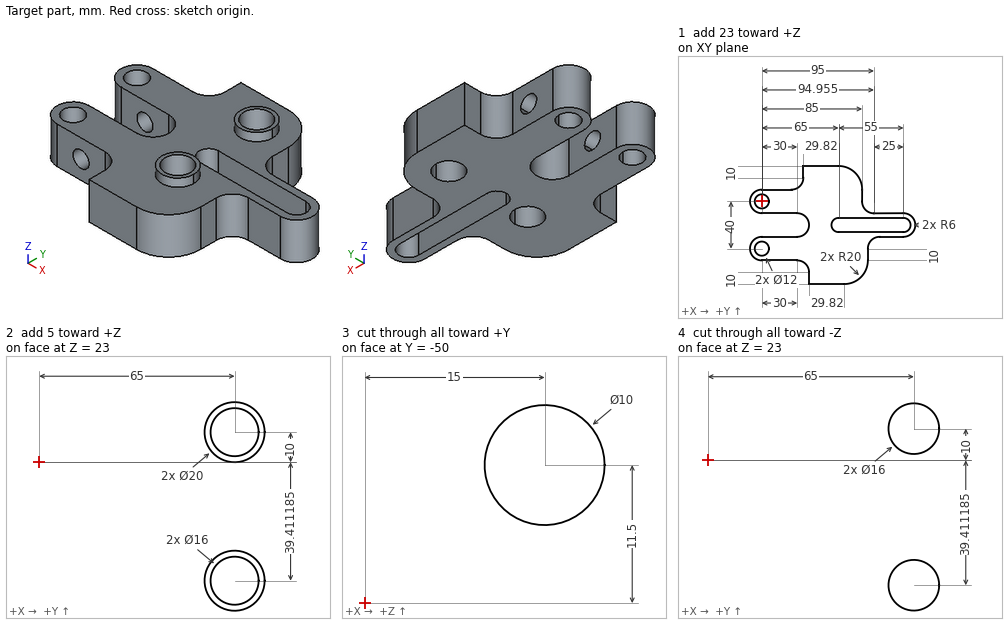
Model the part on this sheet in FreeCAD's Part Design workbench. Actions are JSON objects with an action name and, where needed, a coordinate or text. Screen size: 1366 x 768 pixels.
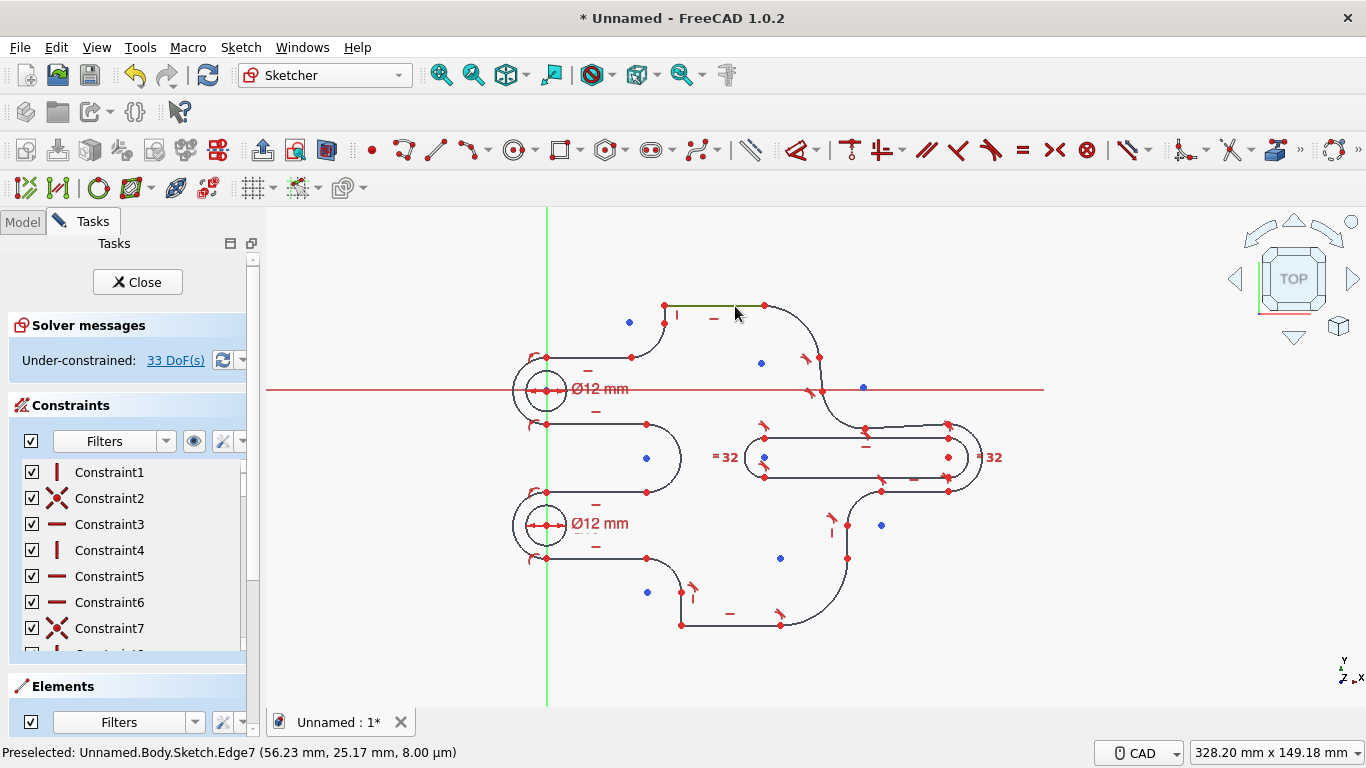
{"action": "left_click", "coordinate": [812, 334]}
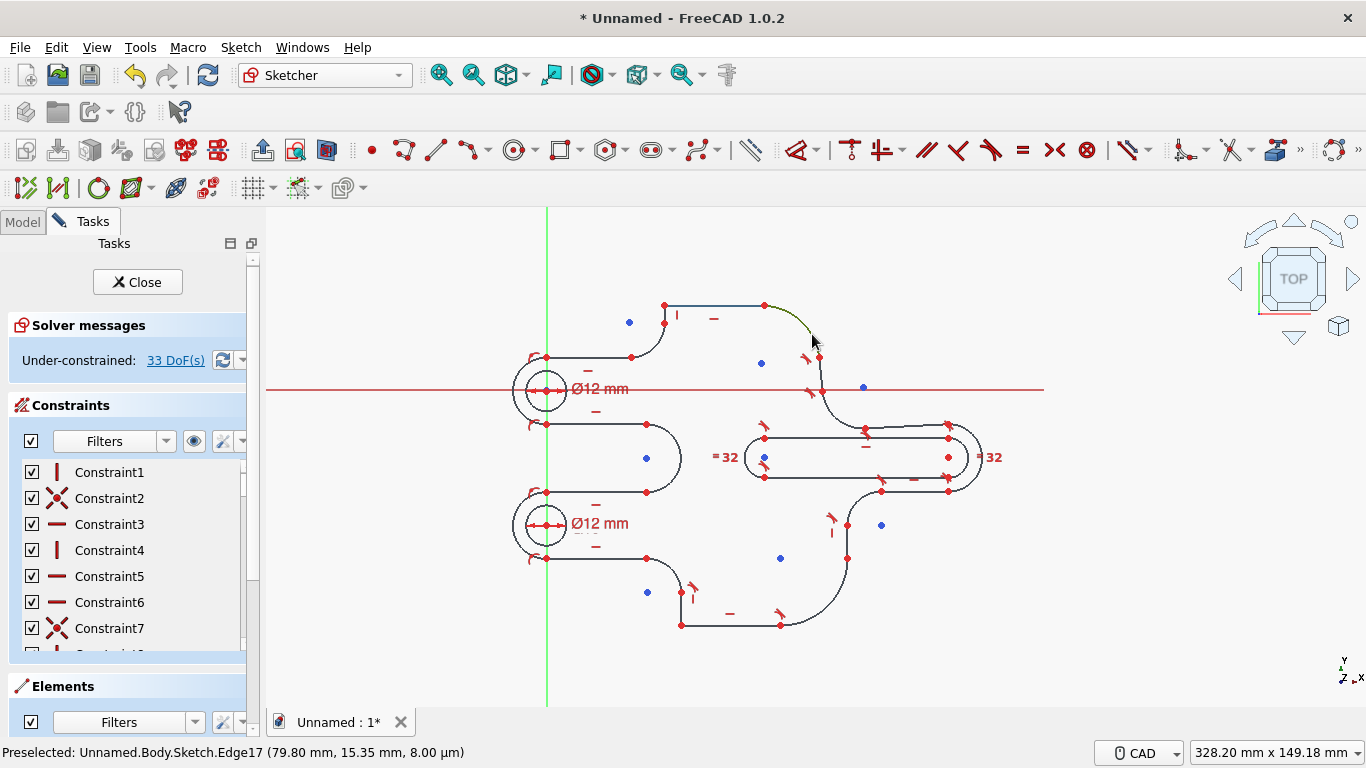
{"action": "left_click", "coordinate": [992, 150]}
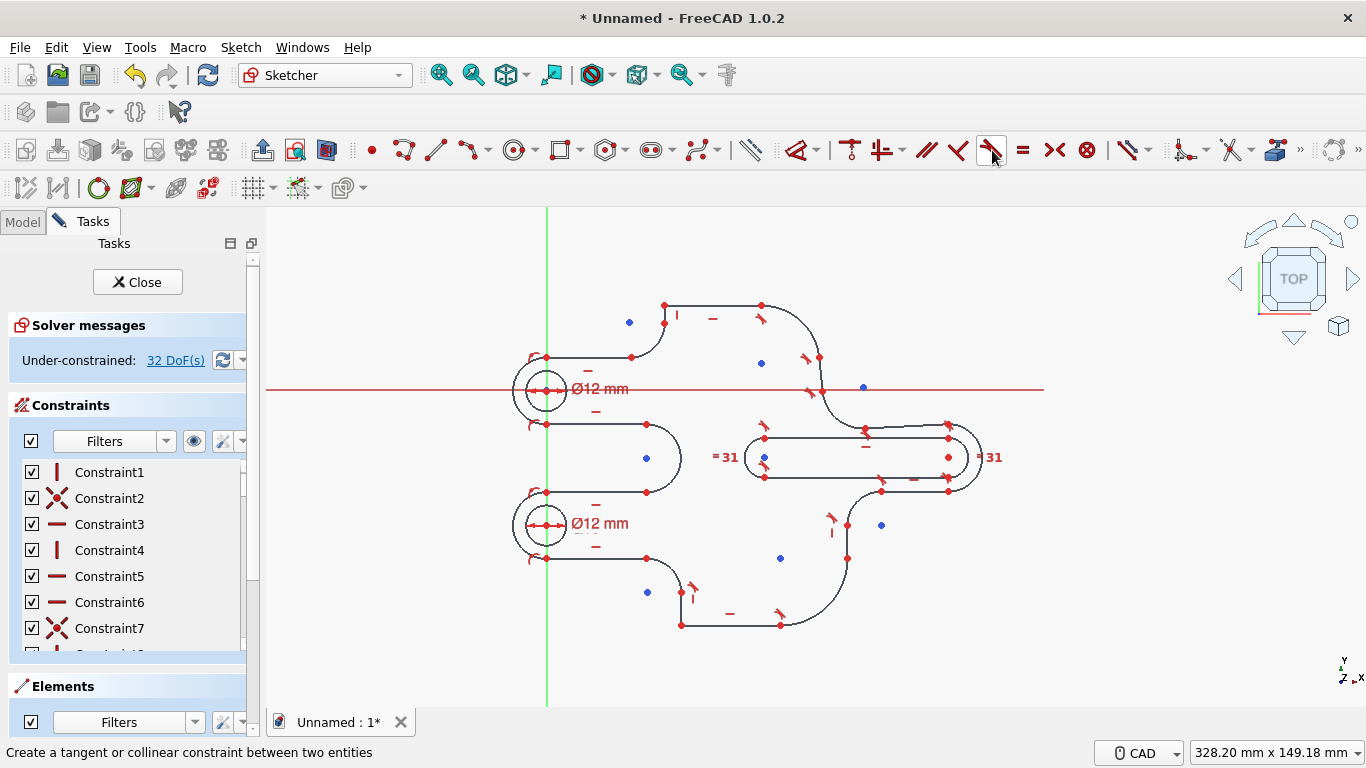
{"action": "scroll", "coordinate": [665, 315], "scroll_direction": "up", "scroll_amount": 3}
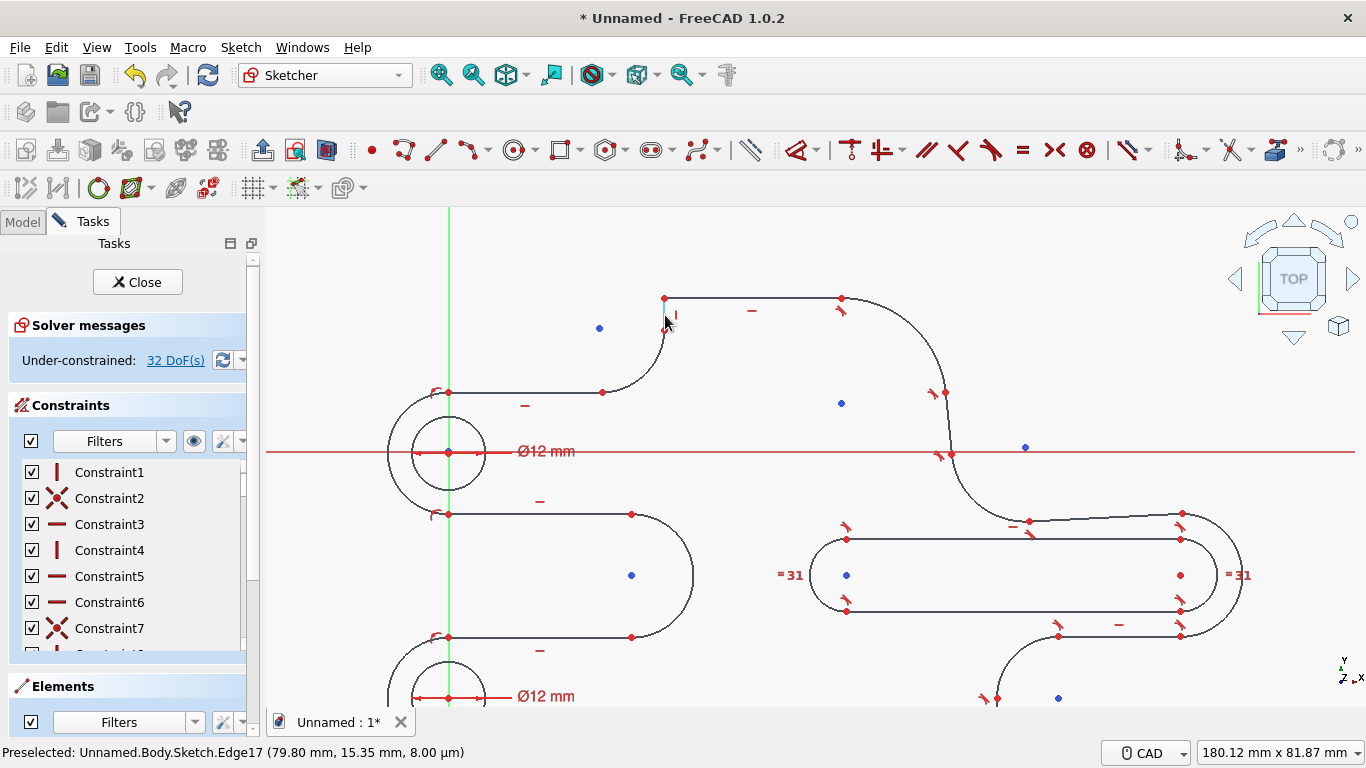
{"action": "left_click", "coordinate": [664, 315]}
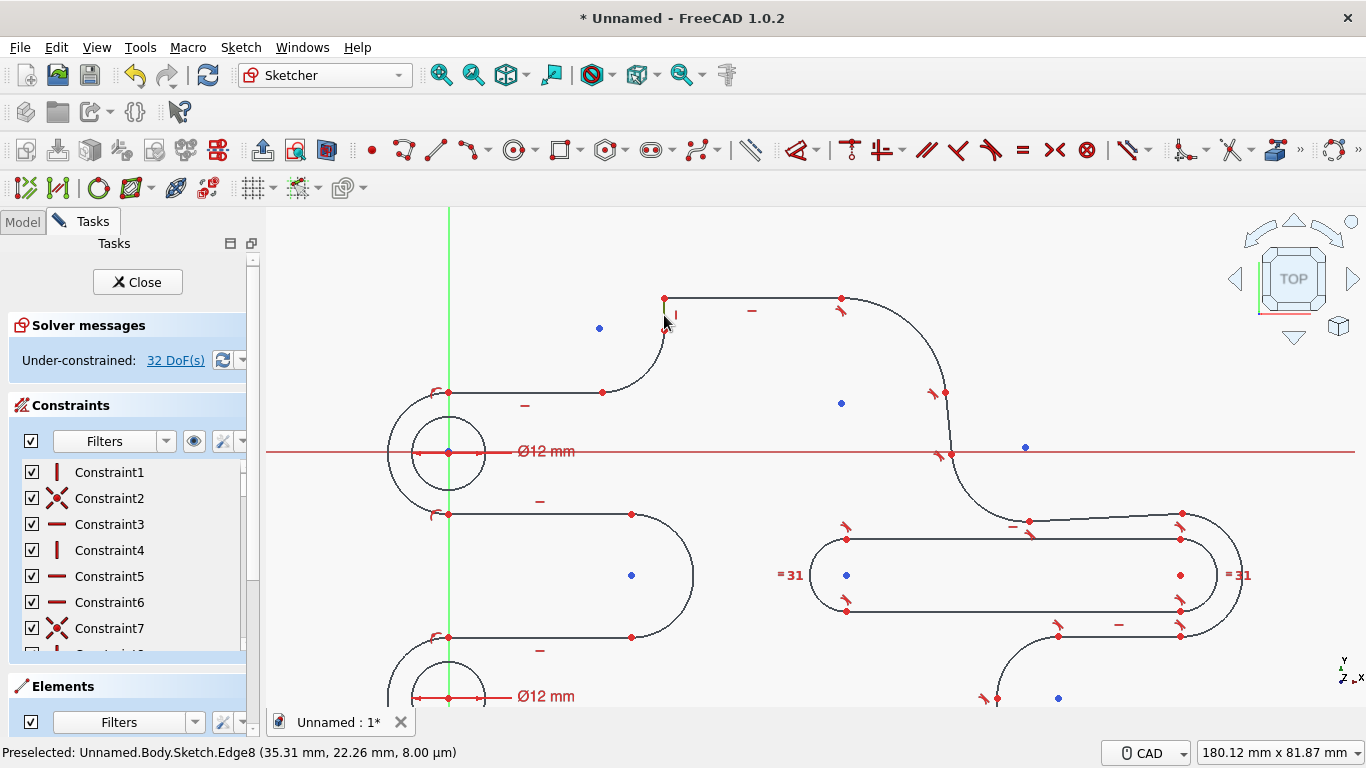
{"action": "left_click", "coordinate": [630, 385]}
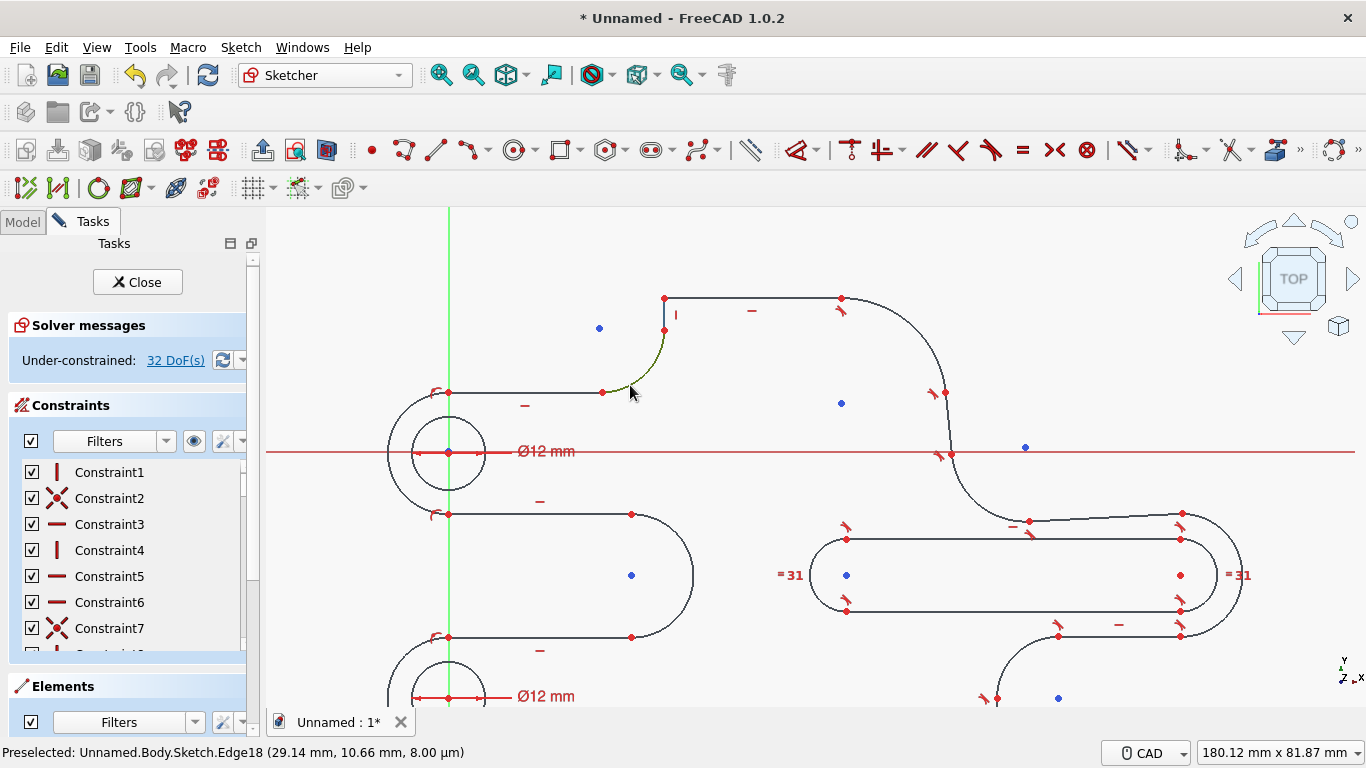
{"action": "left_click", "coordinate": [992, 150]}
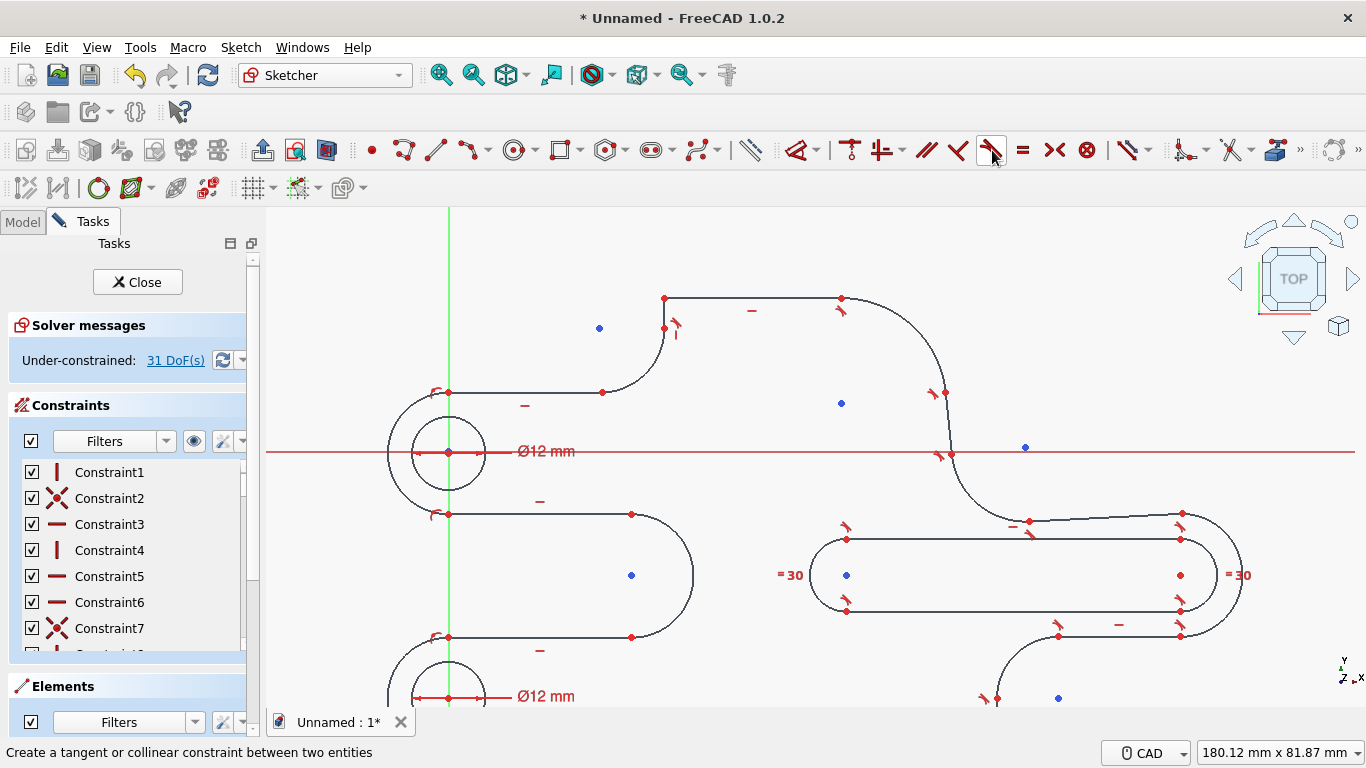
{"action": "left_click", "coordinate": [557, 393]}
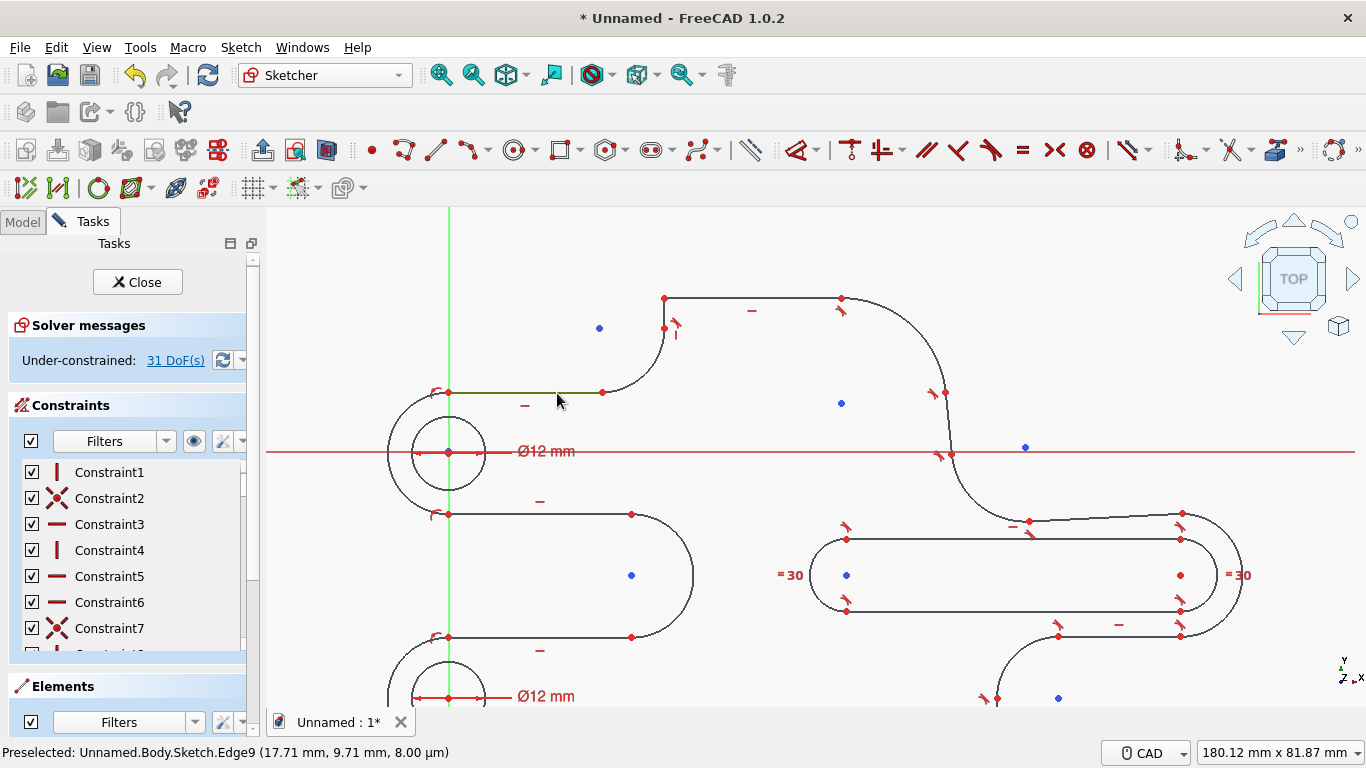
{"action": "left_click", "coordinate": [631, 385]}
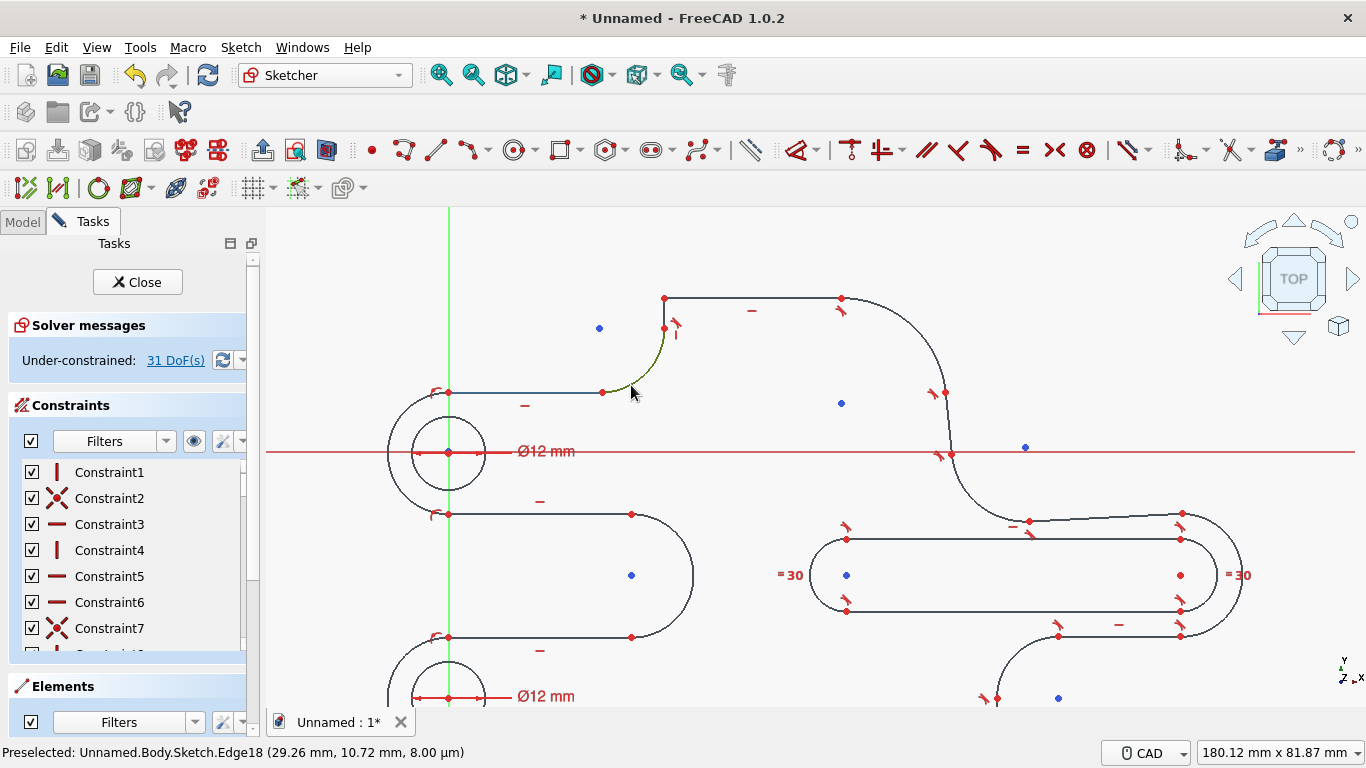
{"action": "key", "text": "t"}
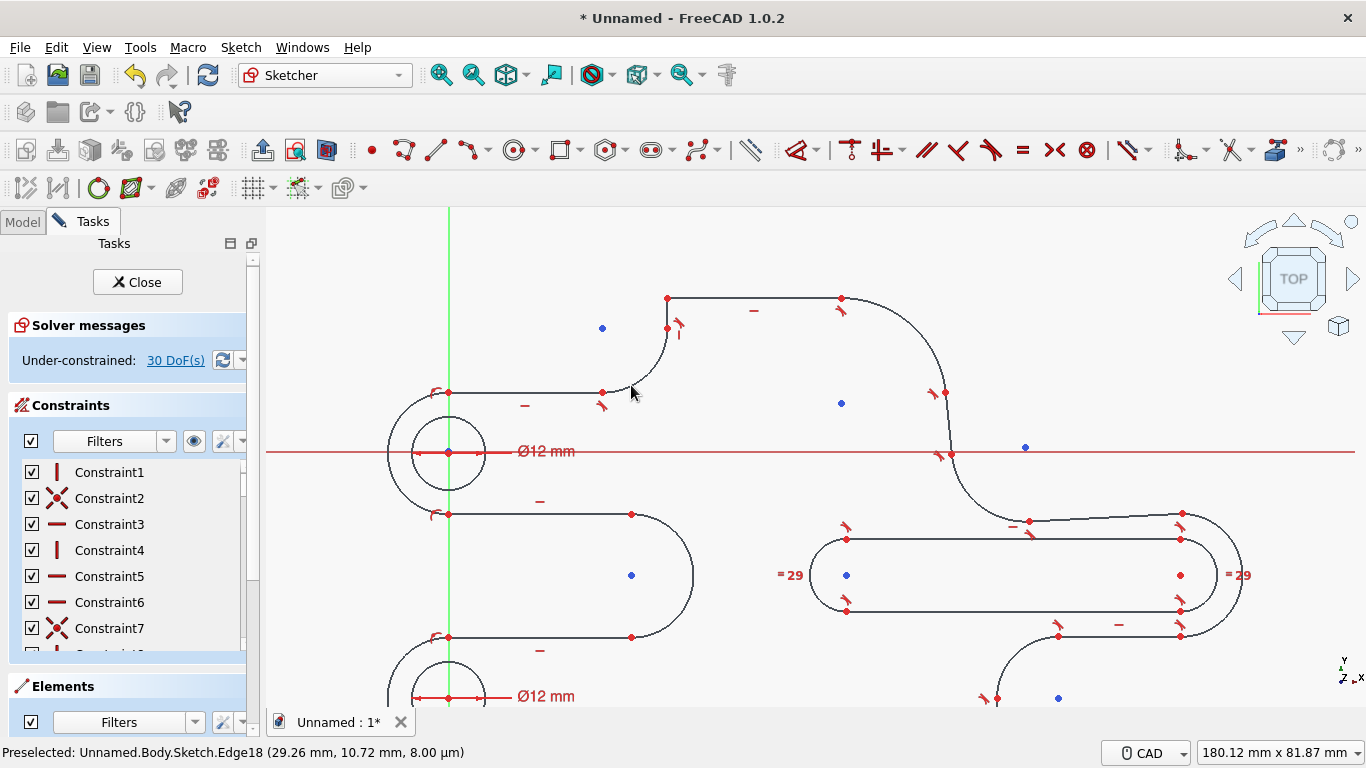
{"action": "left_click", "coordinate": [557, 393]}